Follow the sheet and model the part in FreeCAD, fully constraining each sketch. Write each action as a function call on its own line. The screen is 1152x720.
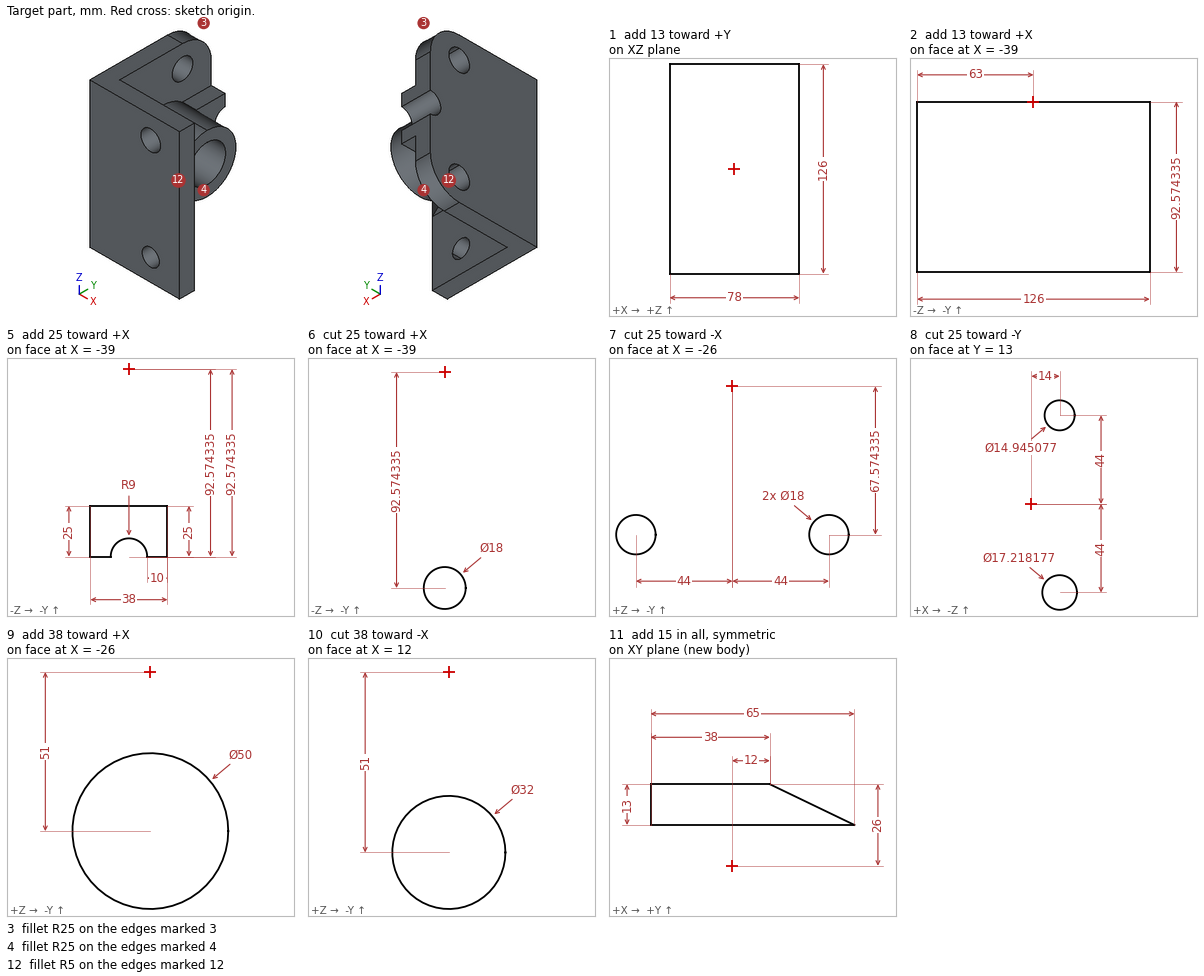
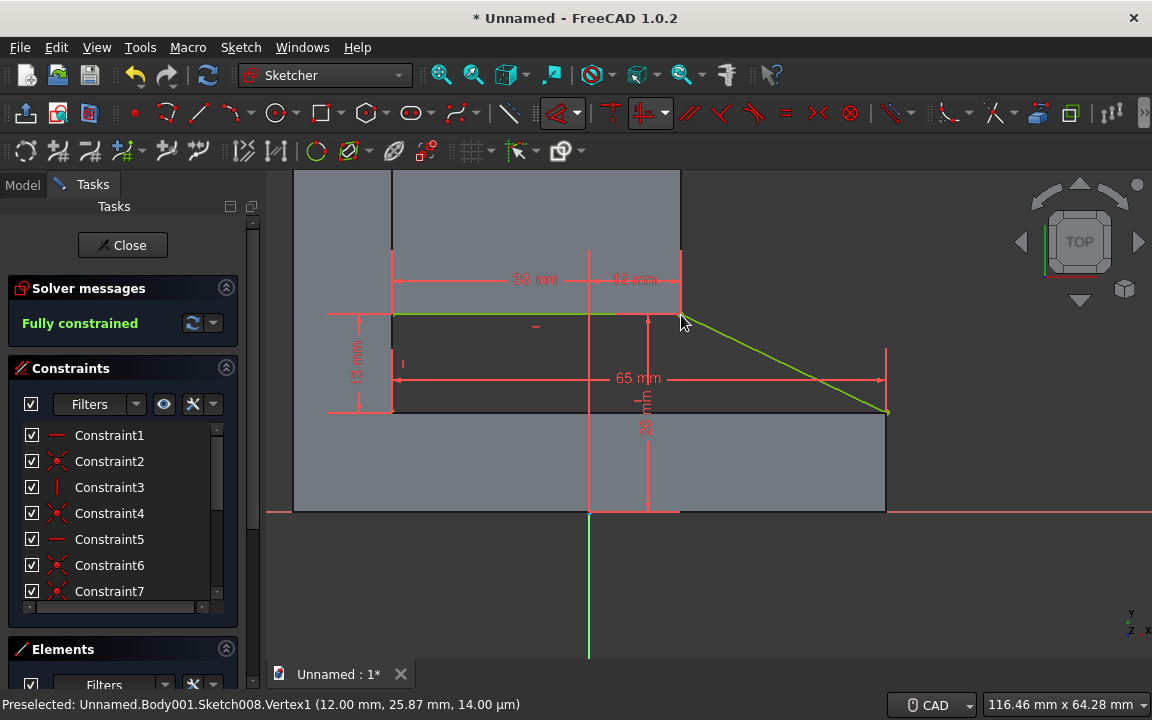
click(123, 245)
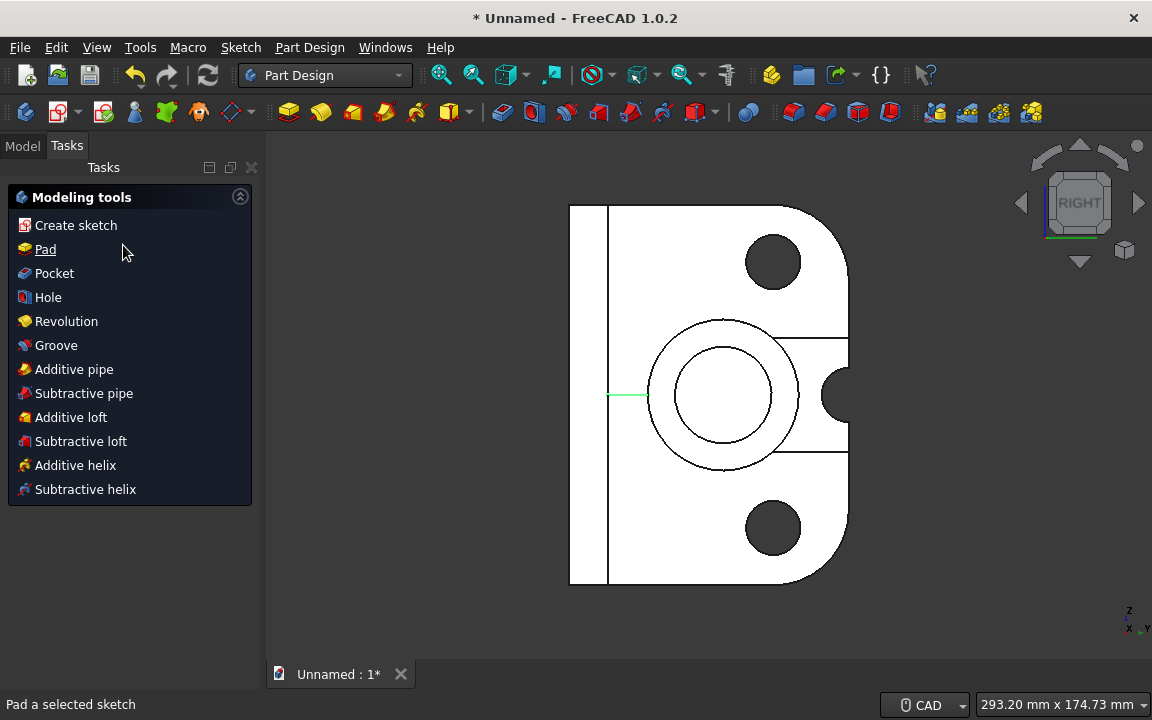
click(290, 112)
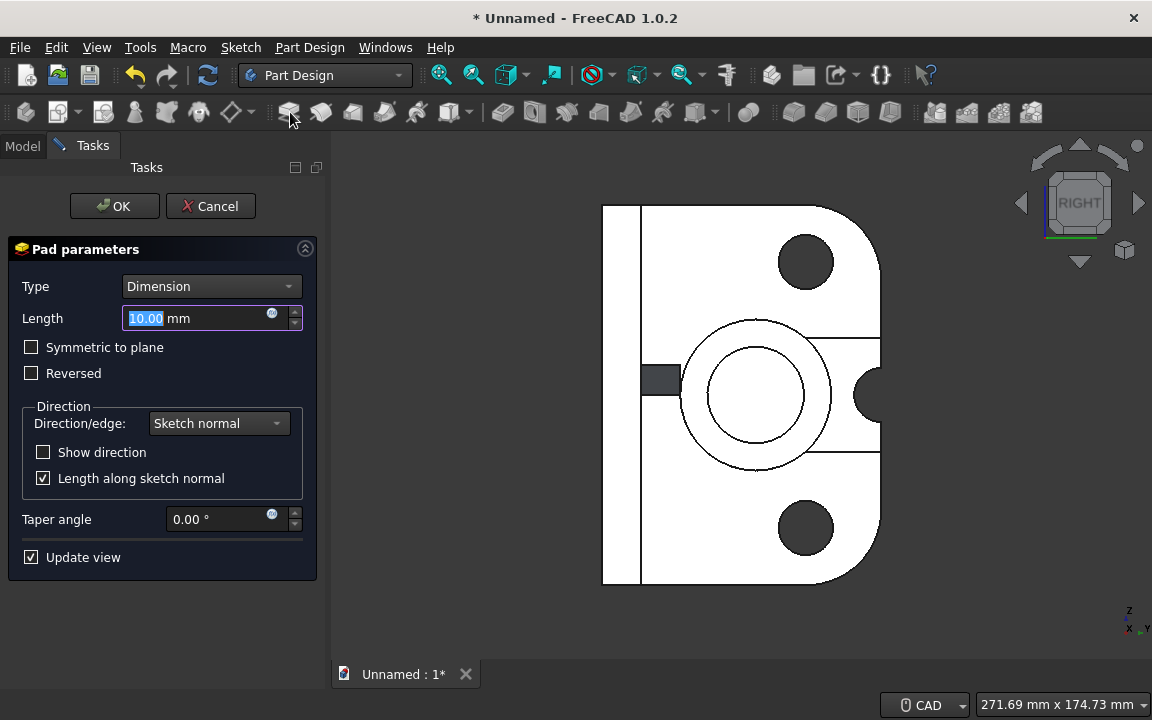
text(15)
key(Tab)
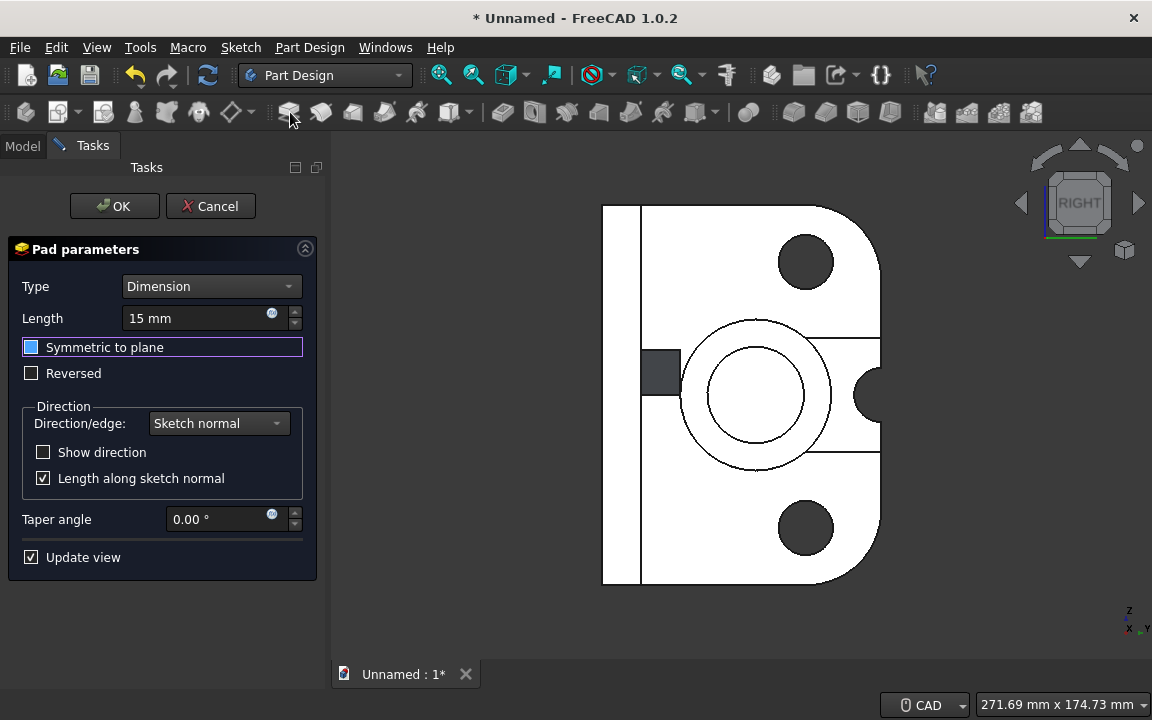
click(30, 347)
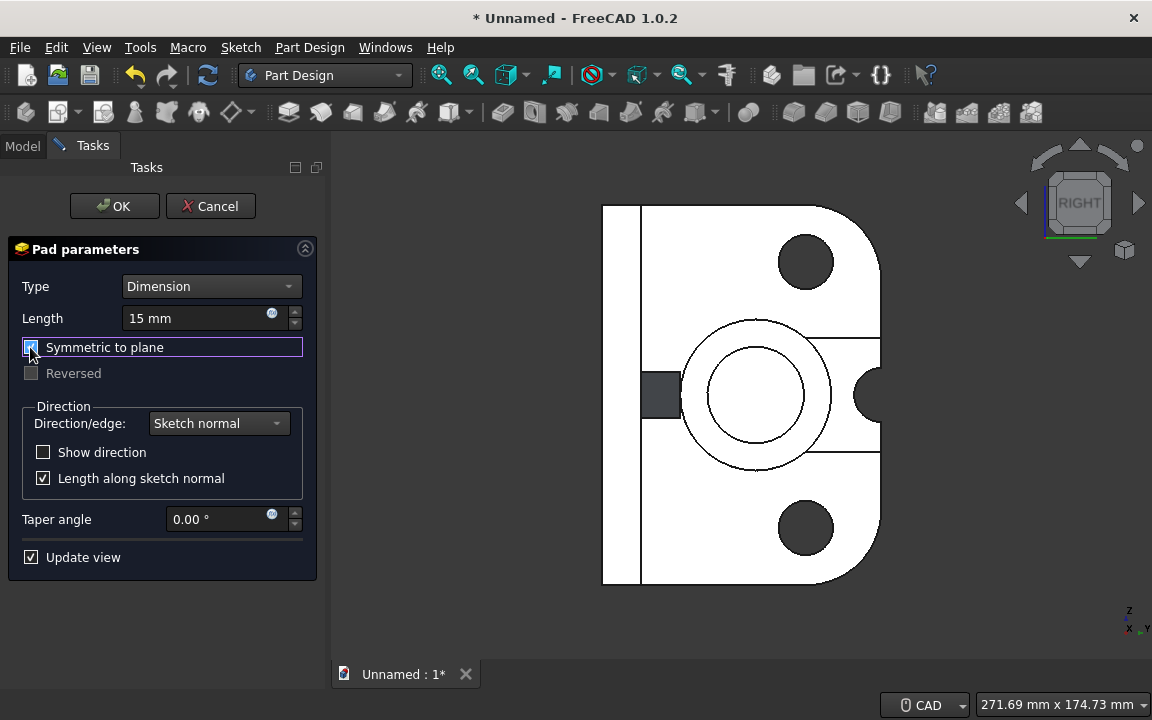
click(115, 206)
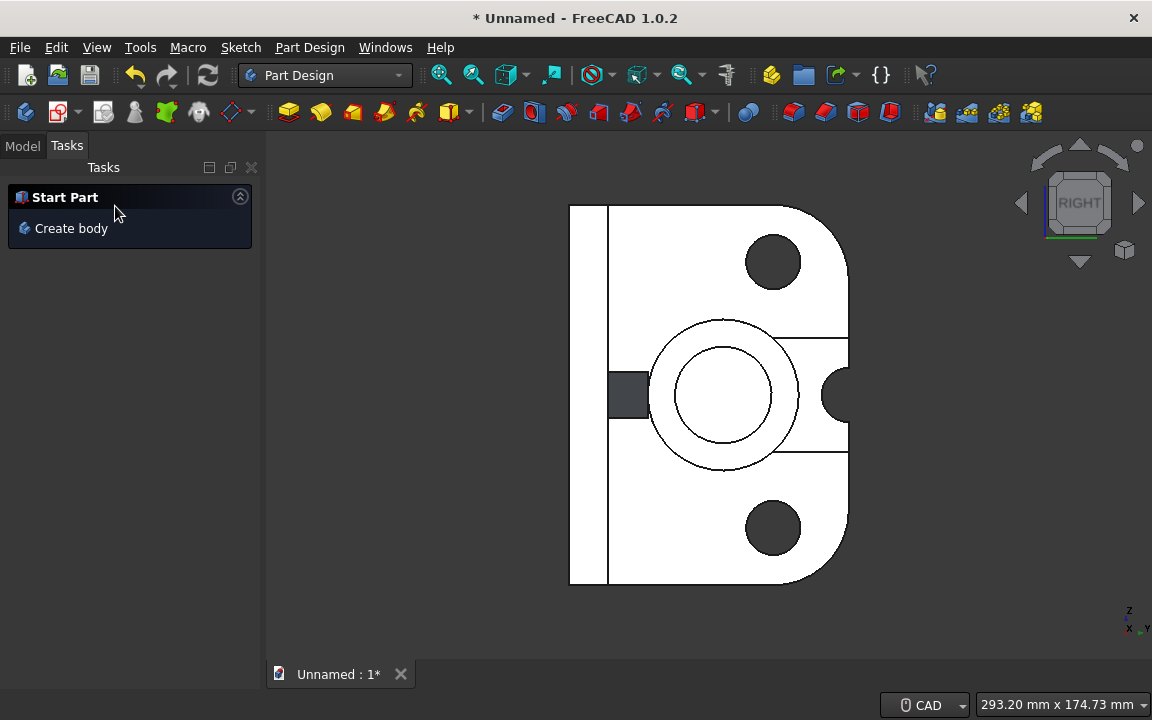
click(442, 76)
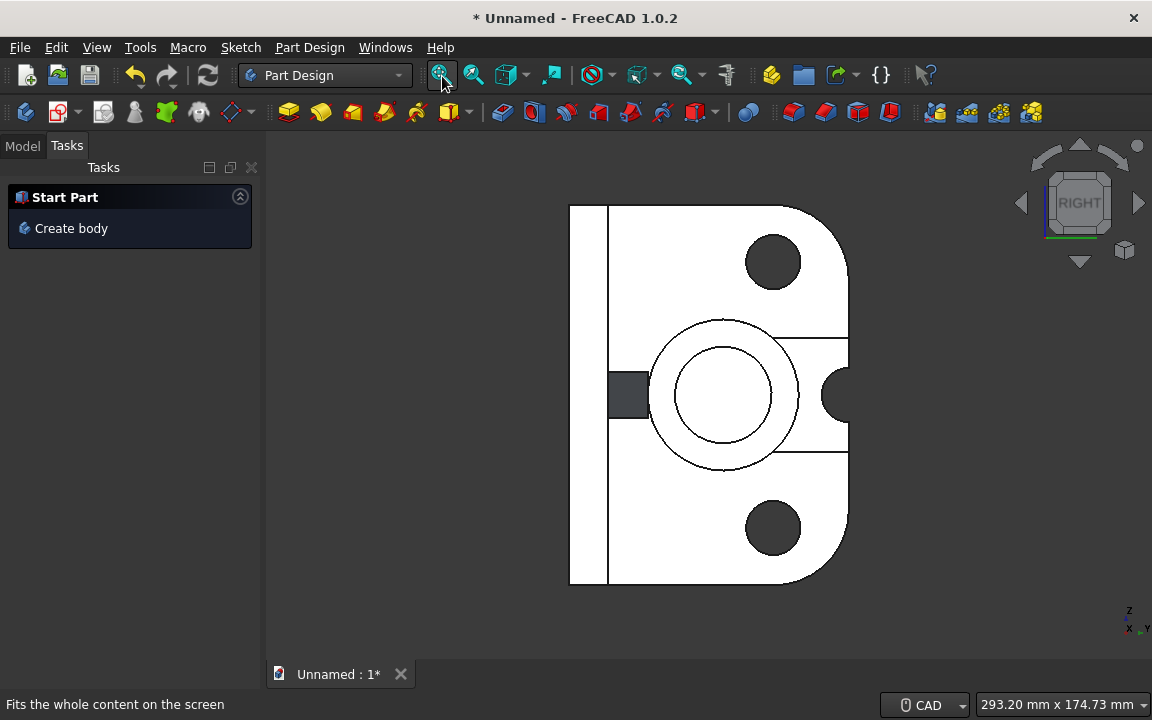
key(0)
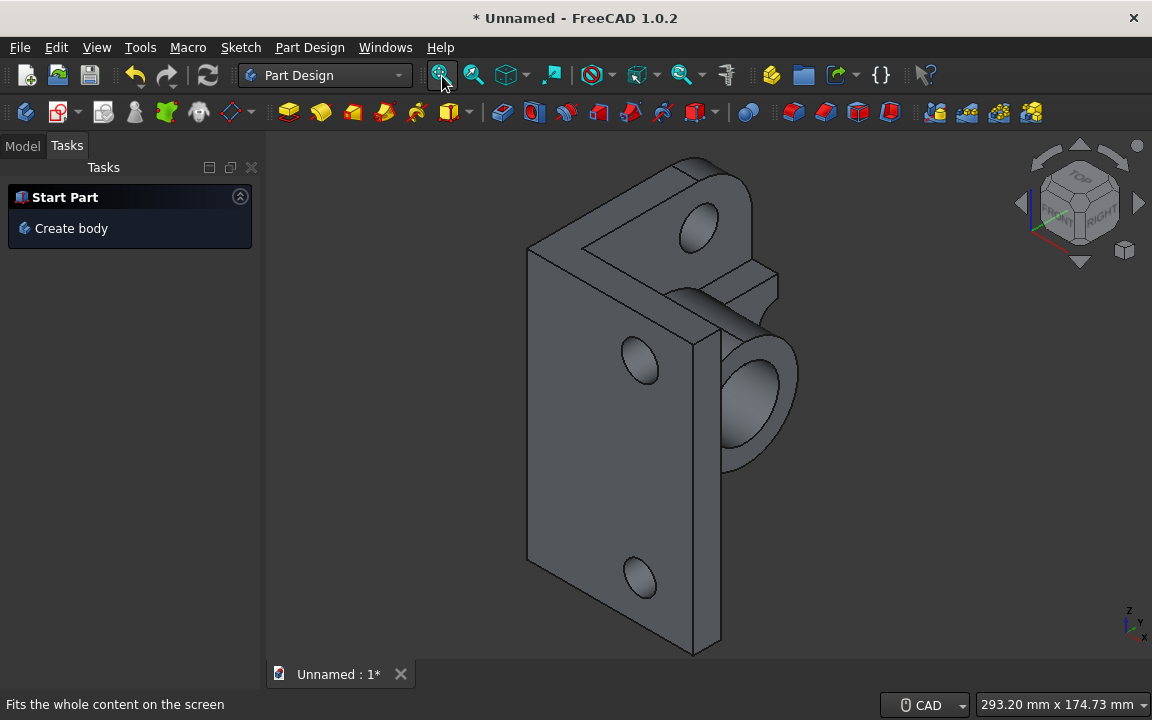
key(v)
key(f)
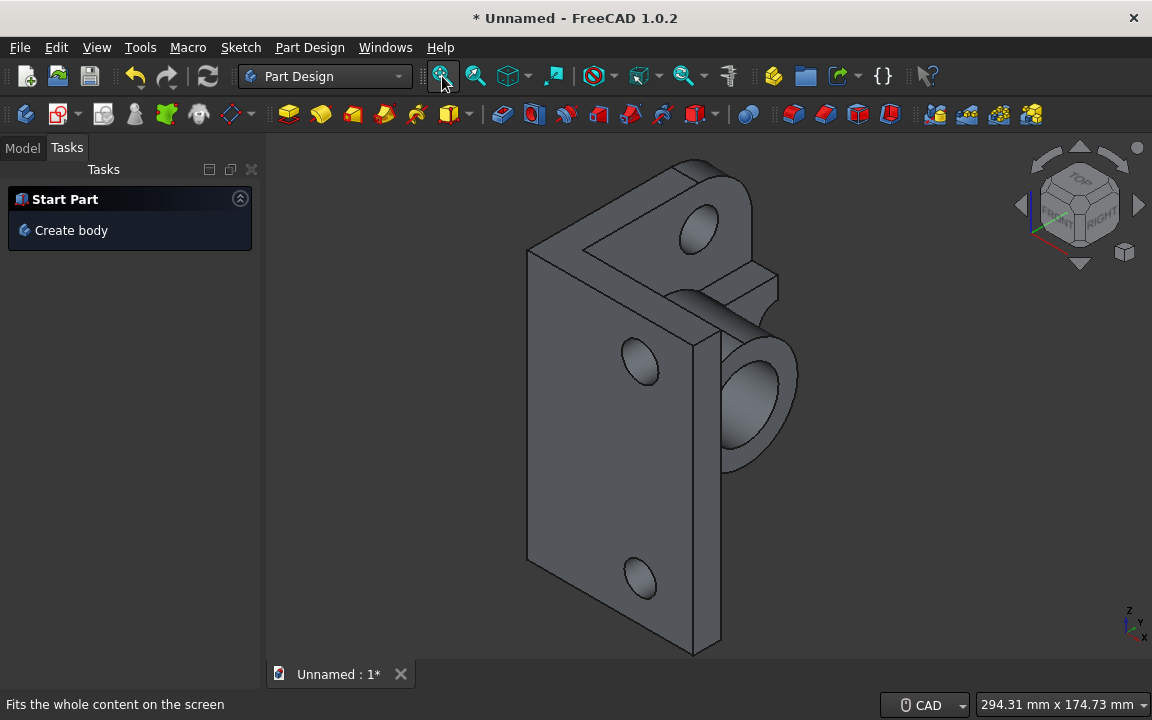
key(2)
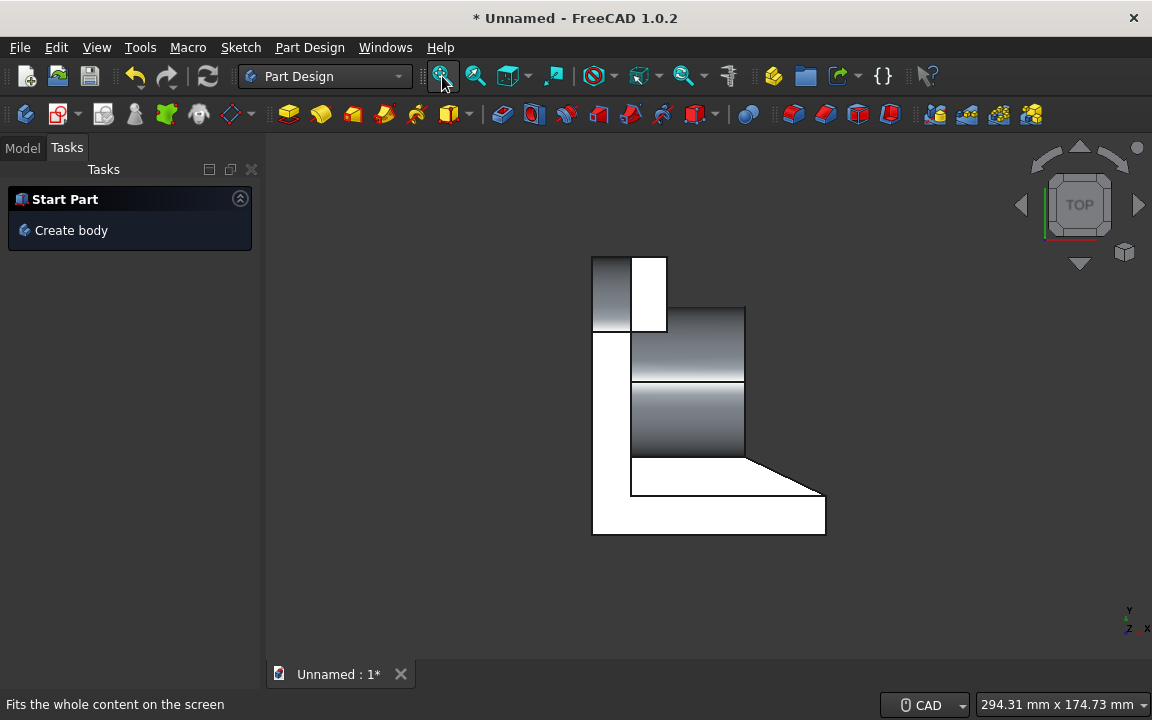
key(v)
key(f)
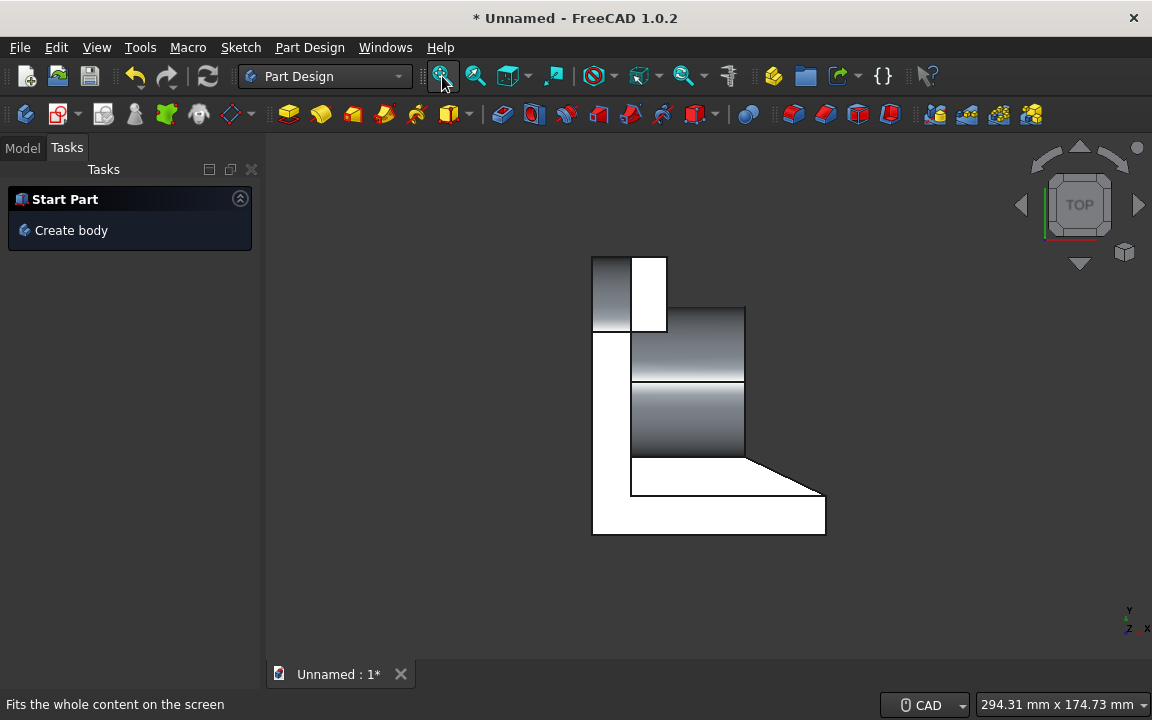
key(1)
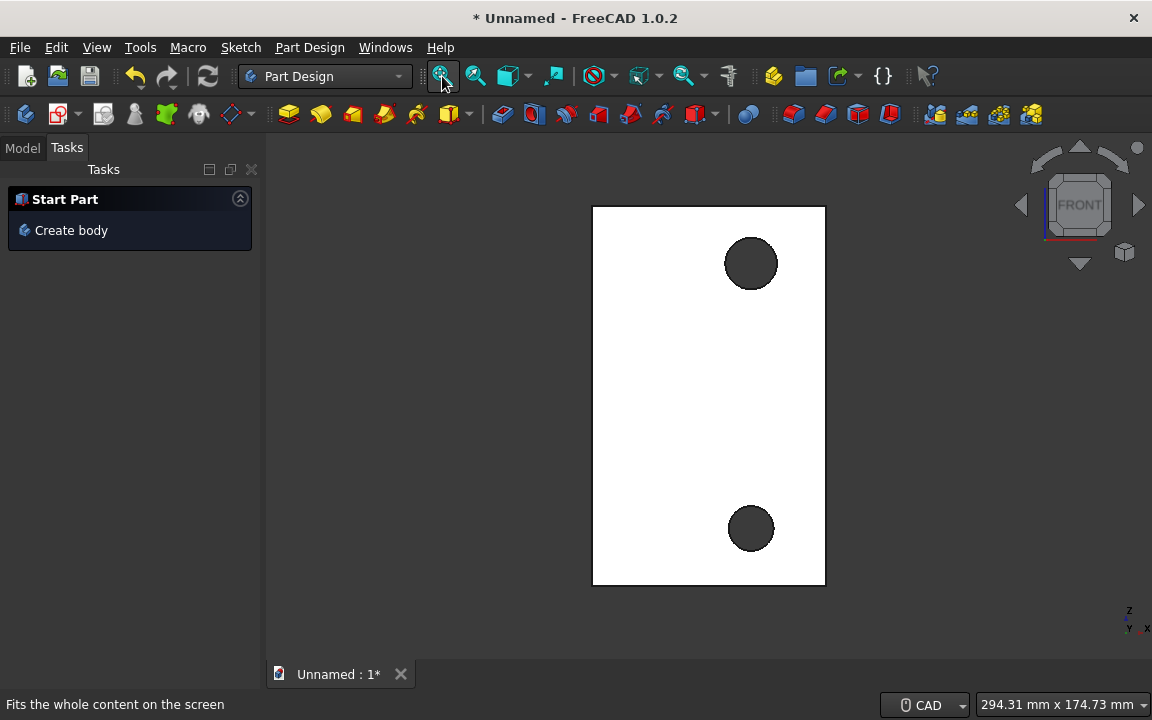
key(v)
key(f)